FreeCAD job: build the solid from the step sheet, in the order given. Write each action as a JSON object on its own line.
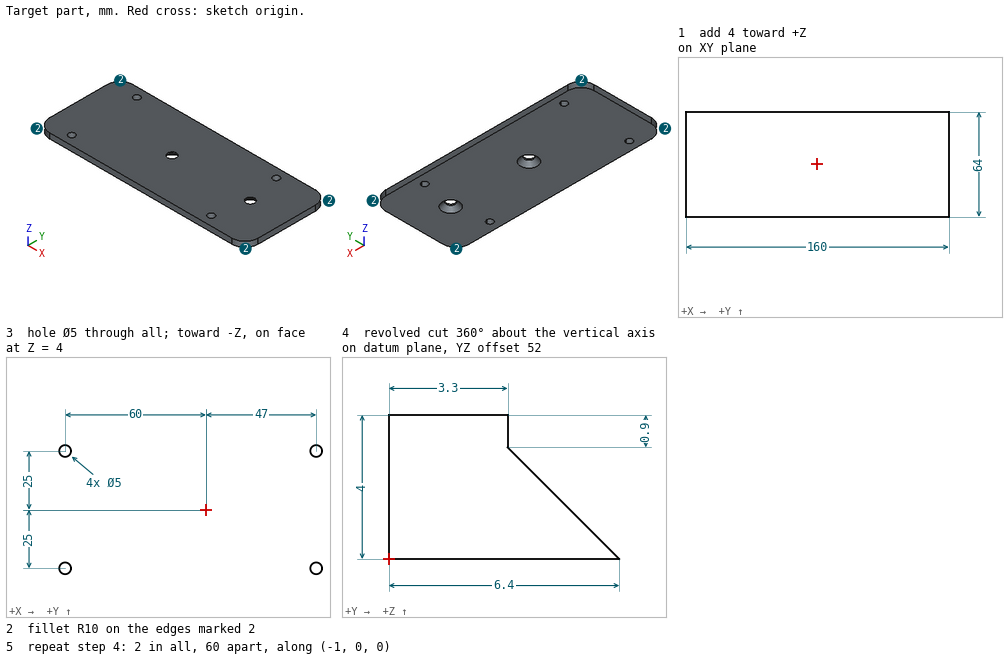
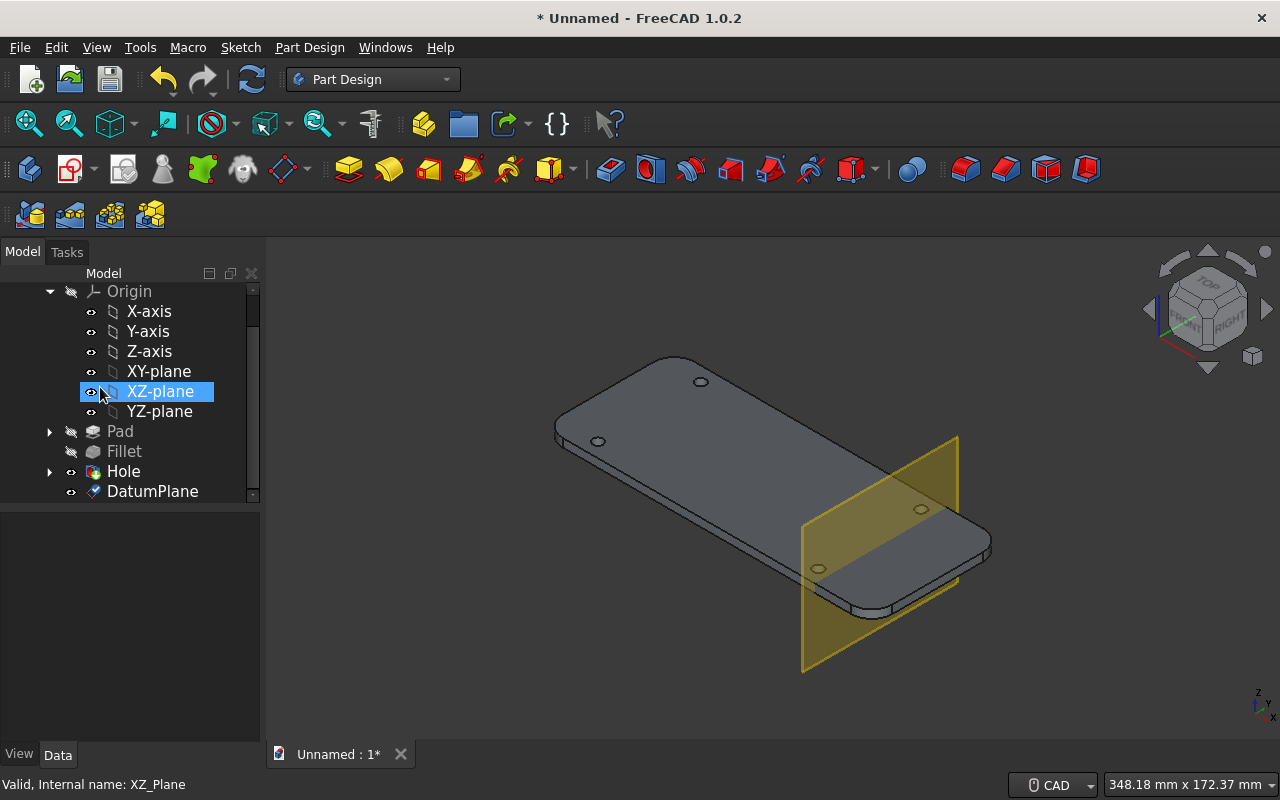
{"action": "left_click", "coordinate": [116, 492]}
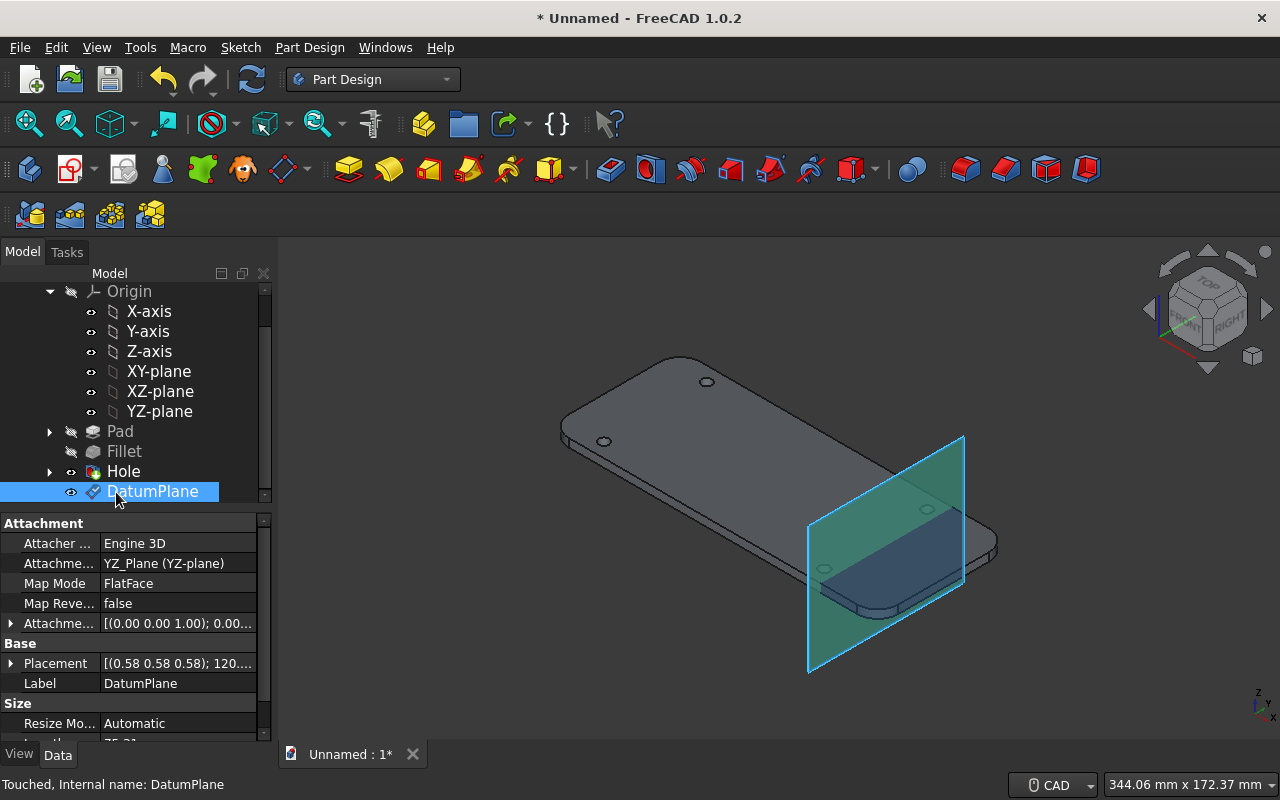
{"action": "left_click", "coordinate": [70, 170]}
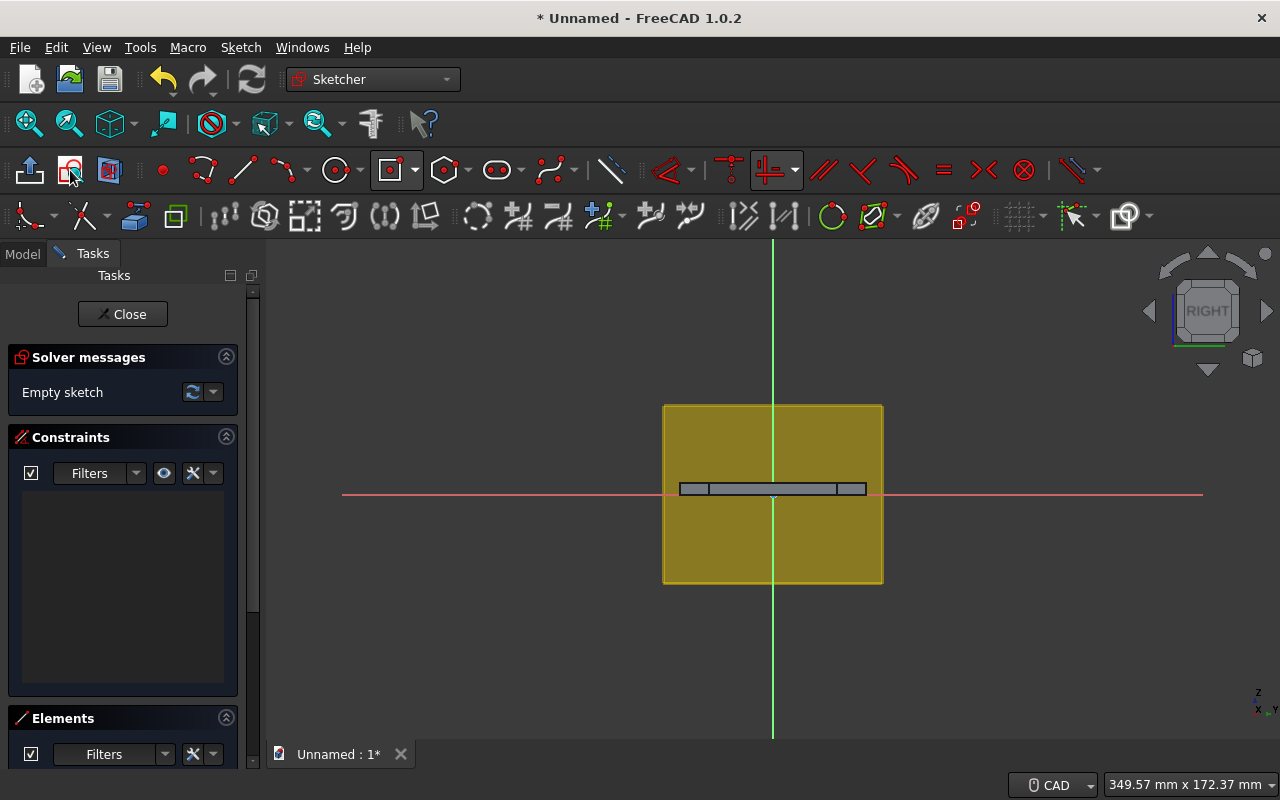
{"action": "left_click", "coordinate": [110, 170]}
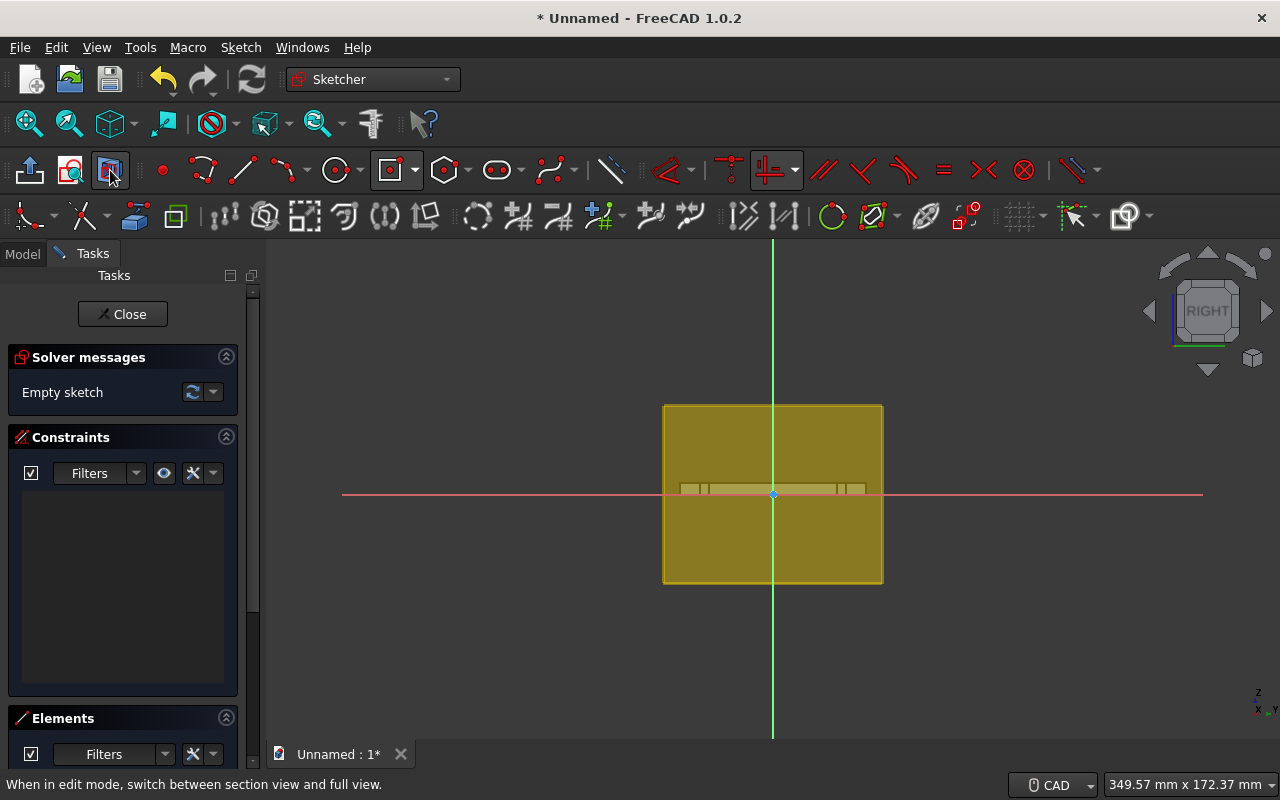
{"action": "scroll", "coordinate": [786, 489], "scroll_direction": "up", "scroll_amount": 15}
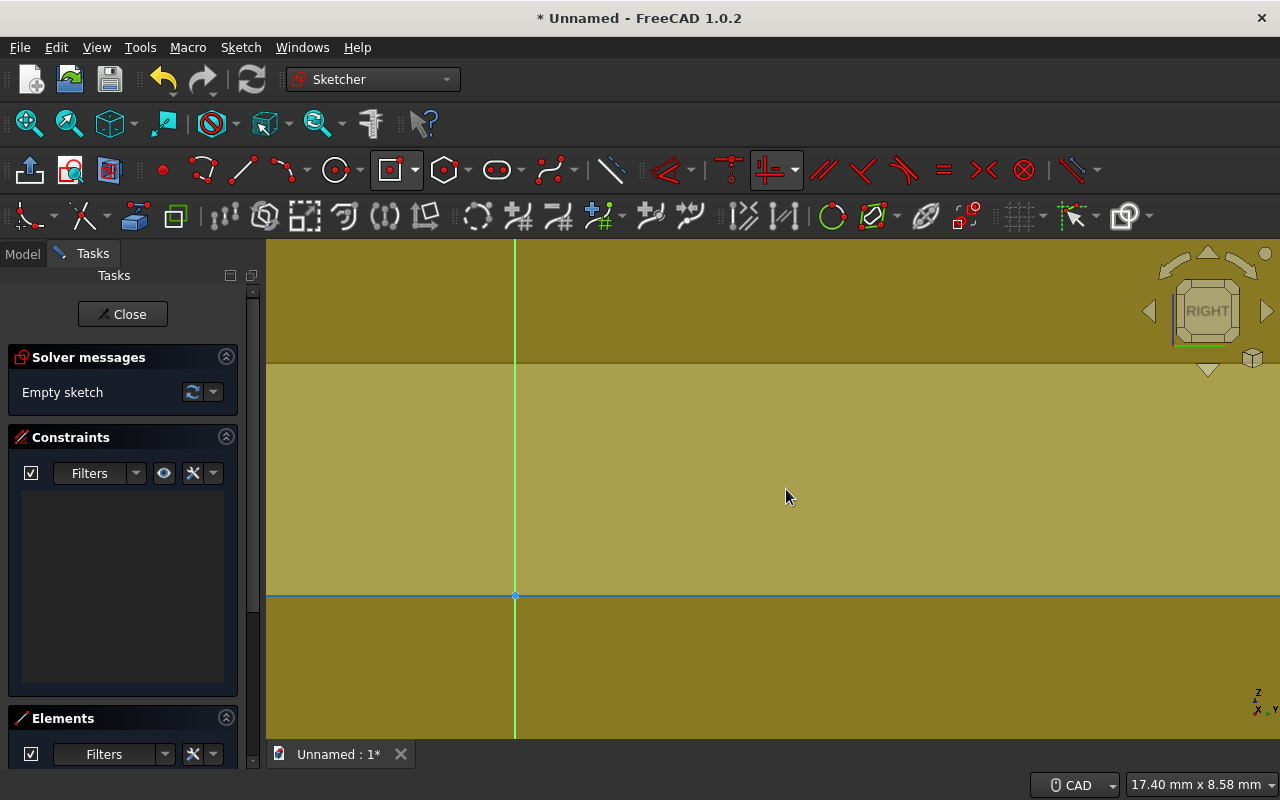
{"action": "left_click", "coordinate": [204, 170]}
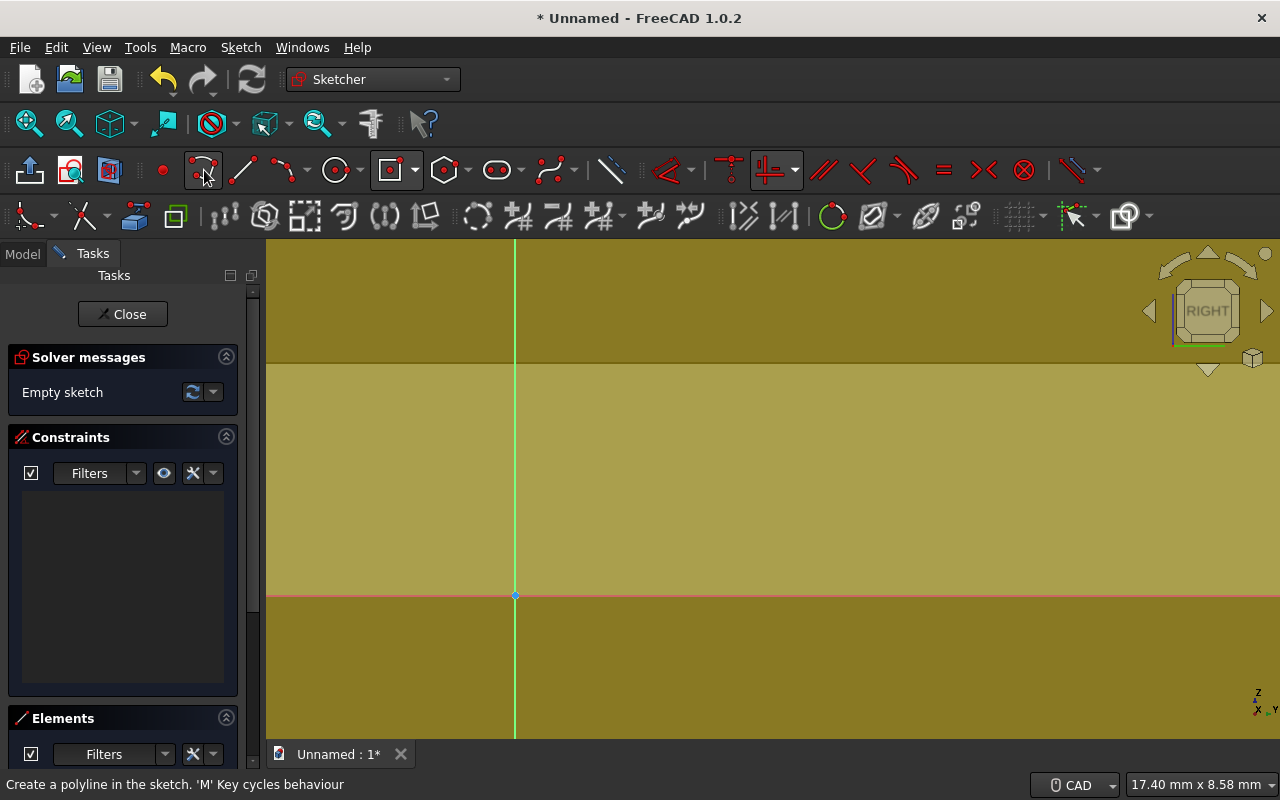
{"action": "left_click", "coordinate": [515, 596]}
{"action": "left_click", "coordinate": [888, 587]}
{"action": "left_click", "coordinate": [707, 415]}
{"action": "left_click", "coordinate": [707, 363]}
{"action": "left_click", "coordinate": [524, 363]}
{"action": "left_click", "coordinate": [515, 596]}
{"action": "key", "text": "Escape"}
{"action": "key", "text": "Escape"}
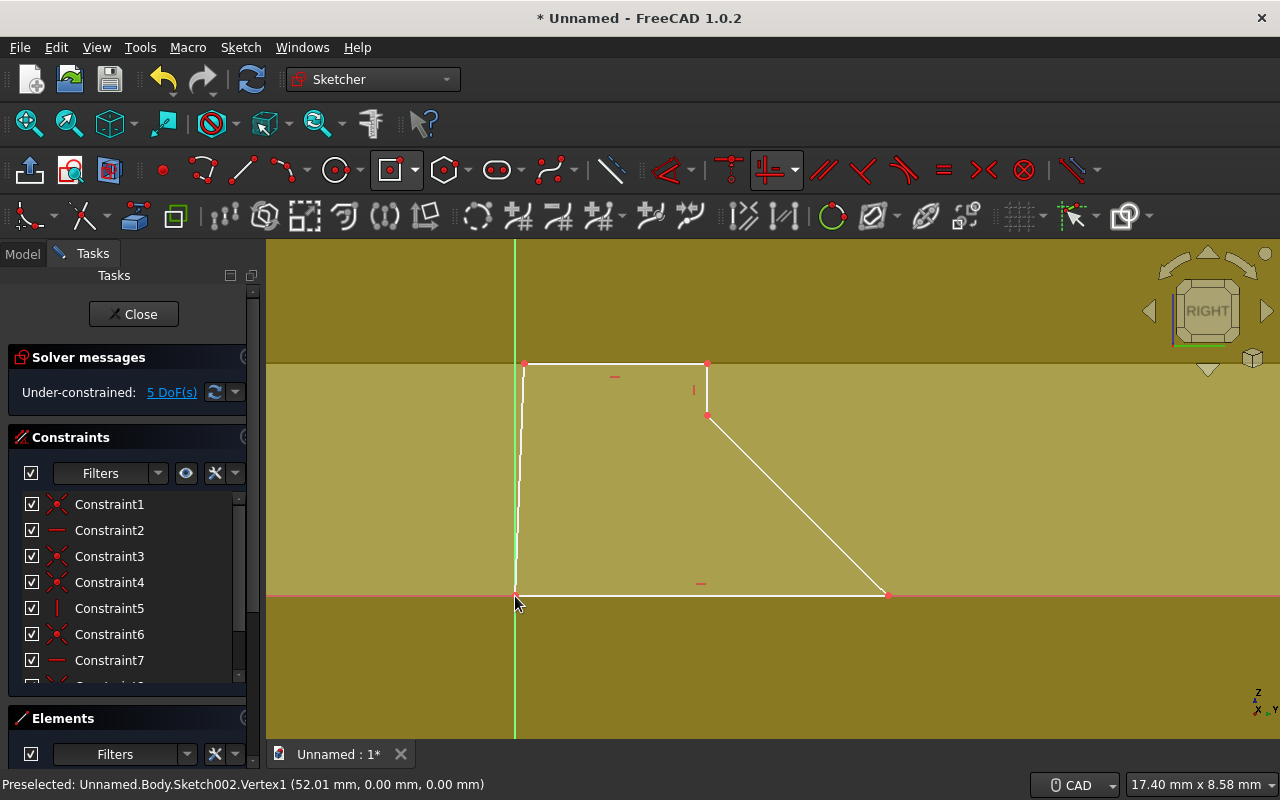
{"action": "left_click", "coordinate": [518, 526]}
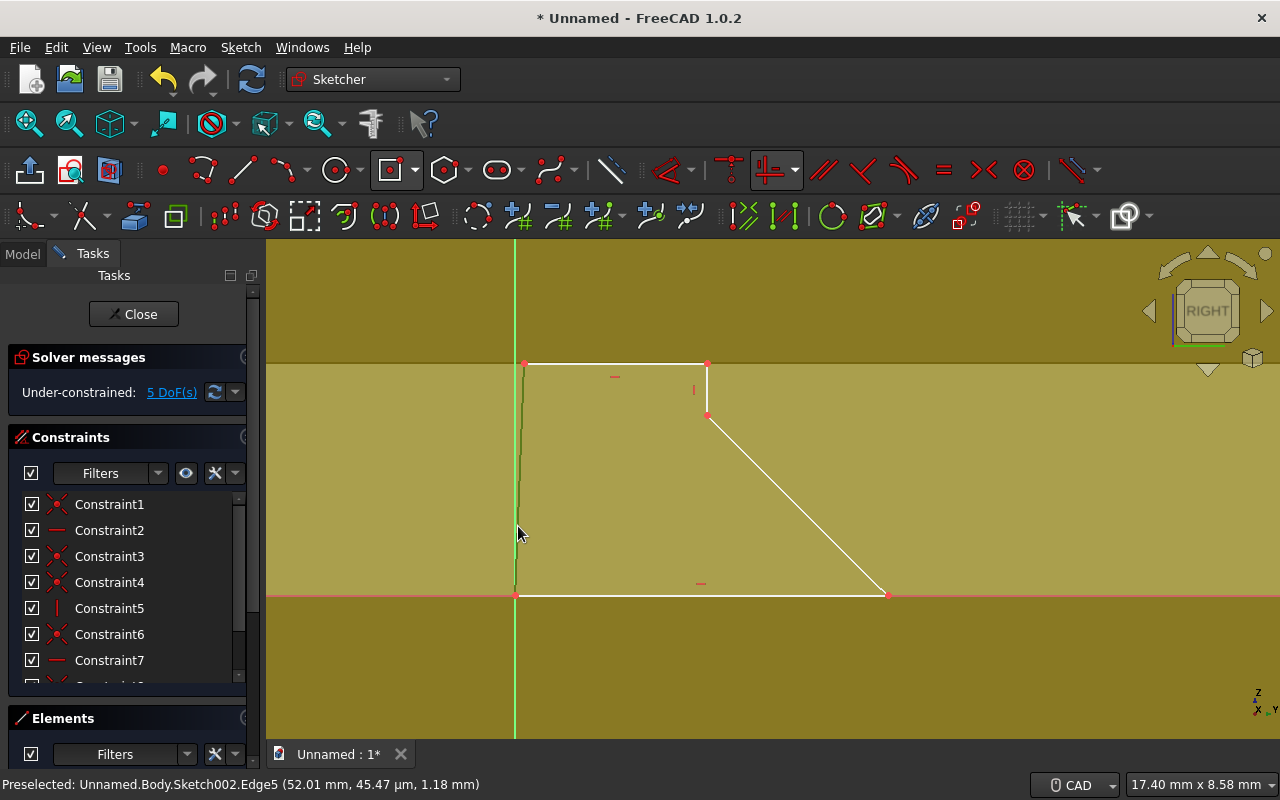
{"action": "left_click", "coordinate": [798, 170]}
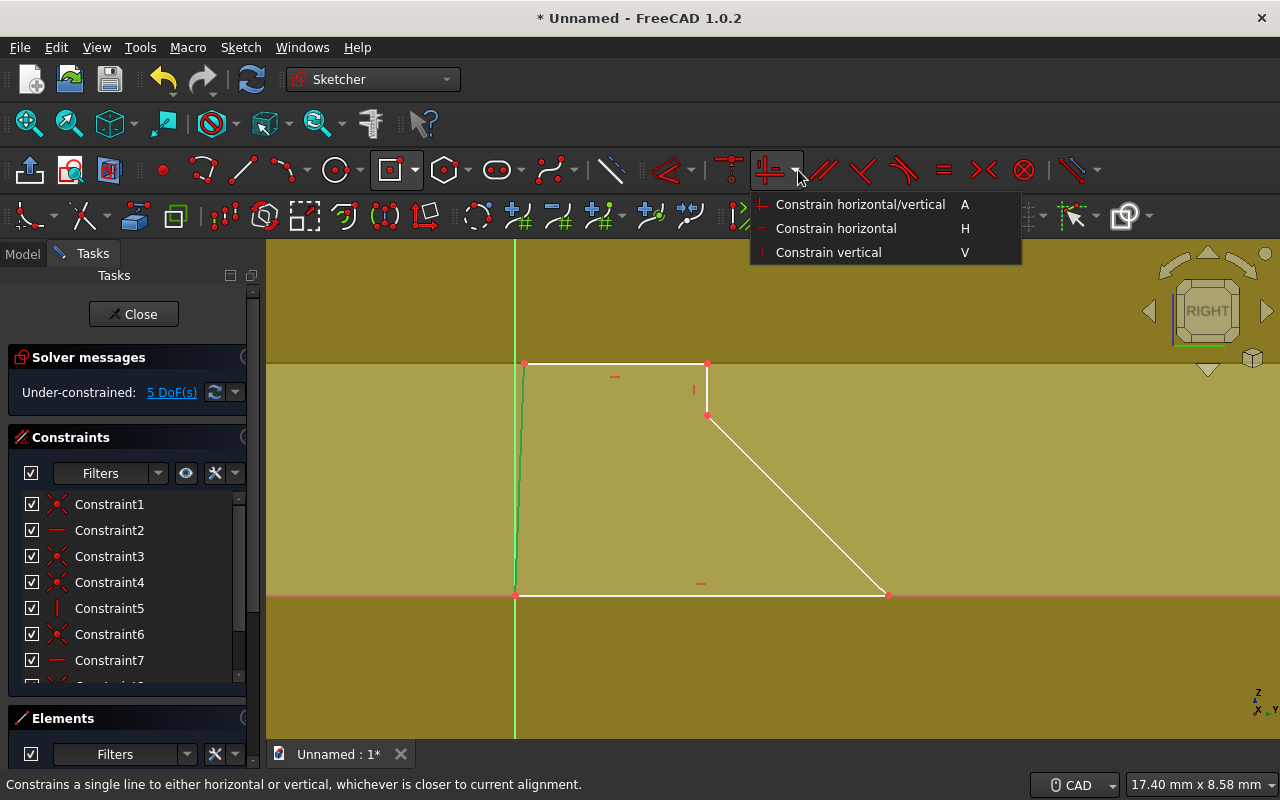
{"action": "left_click", "coordinate": [886, 252]}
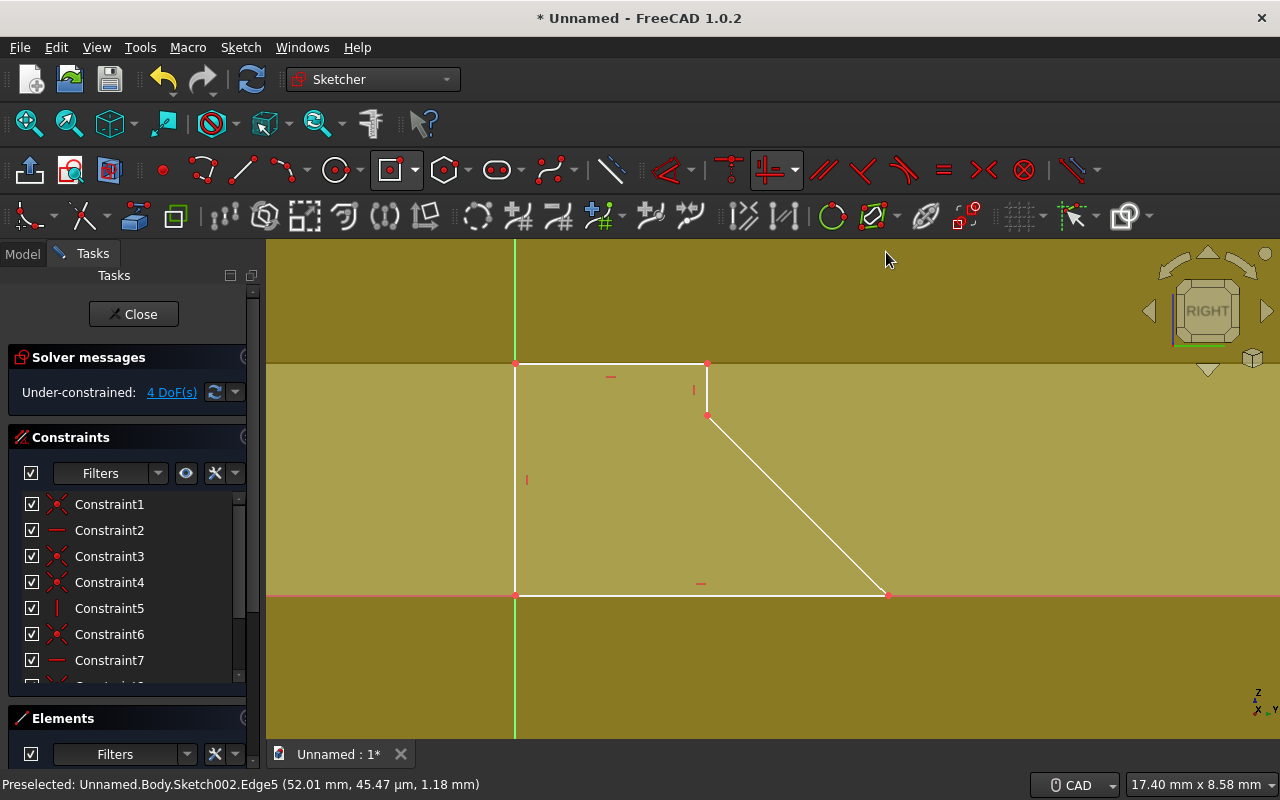
{"action": "left_click", "coordinate": [666, 170]}